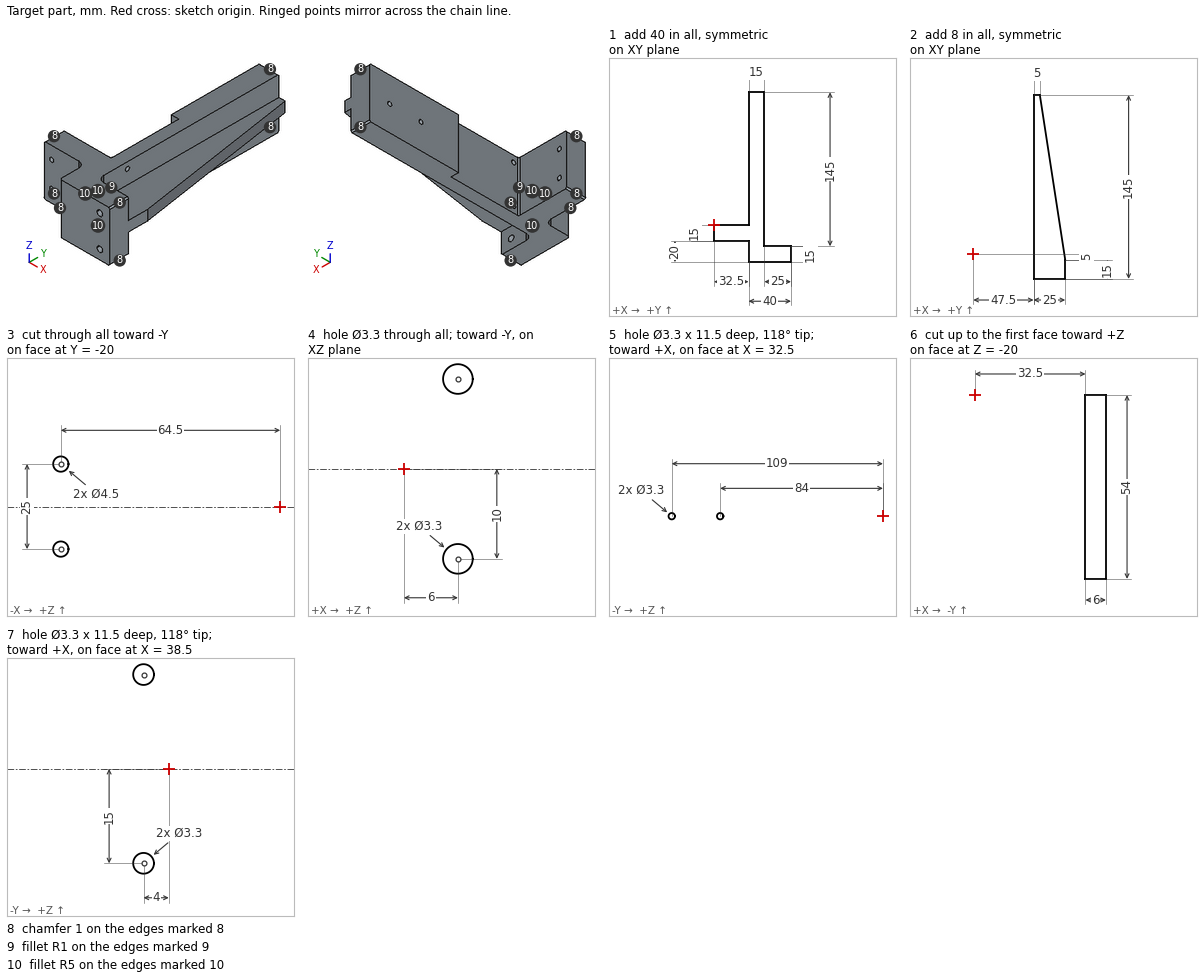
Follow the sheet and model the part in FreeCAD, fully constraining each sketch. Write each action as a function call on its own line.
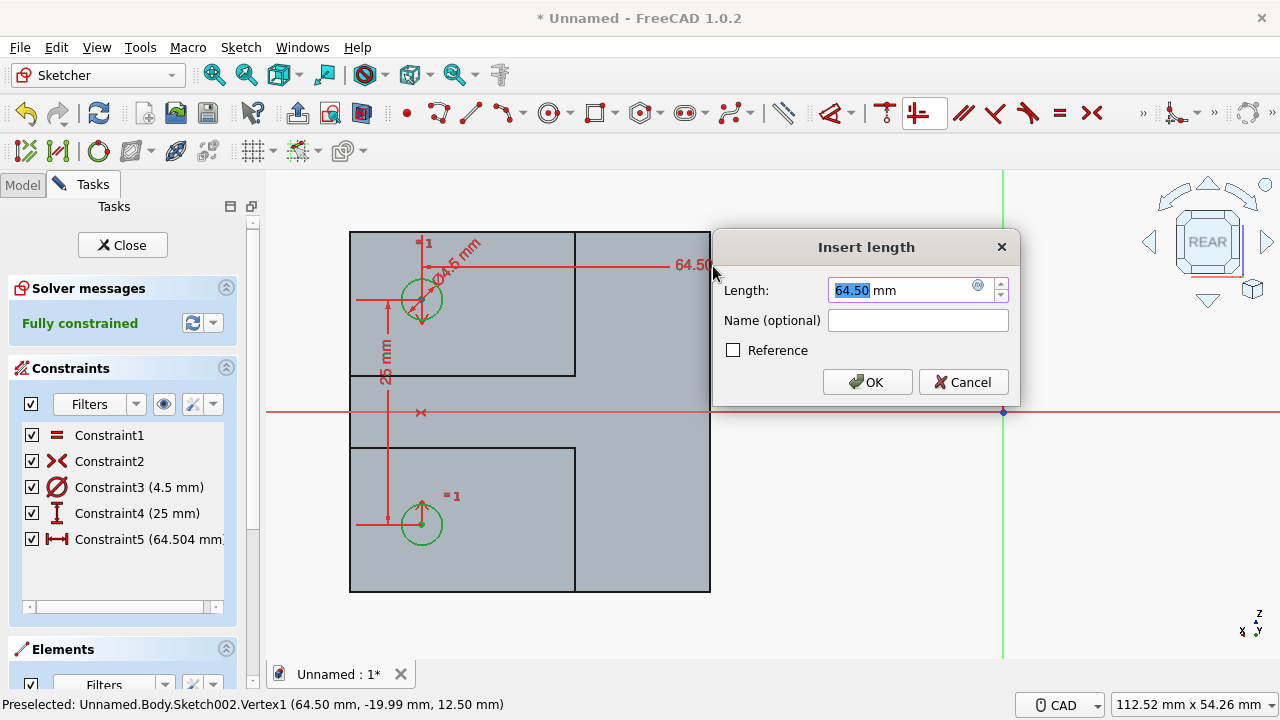
text(64.5)
key(Return)
key(Escape)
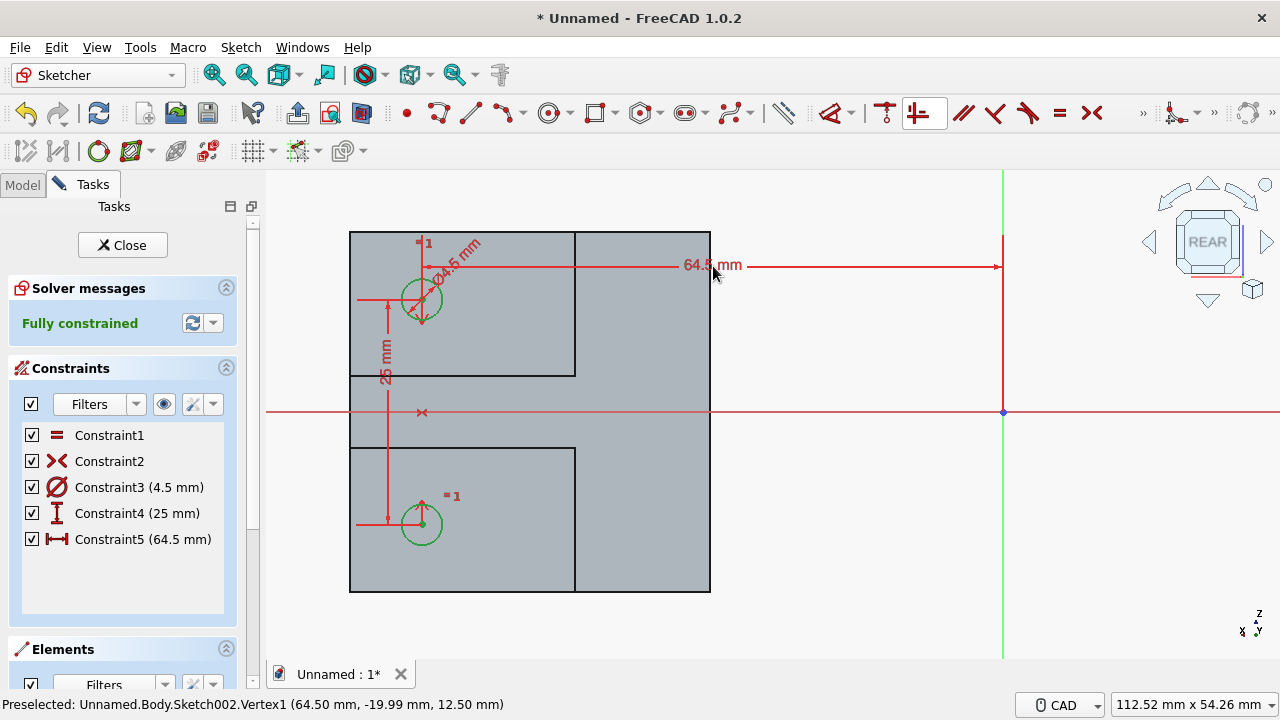
click(123, 245)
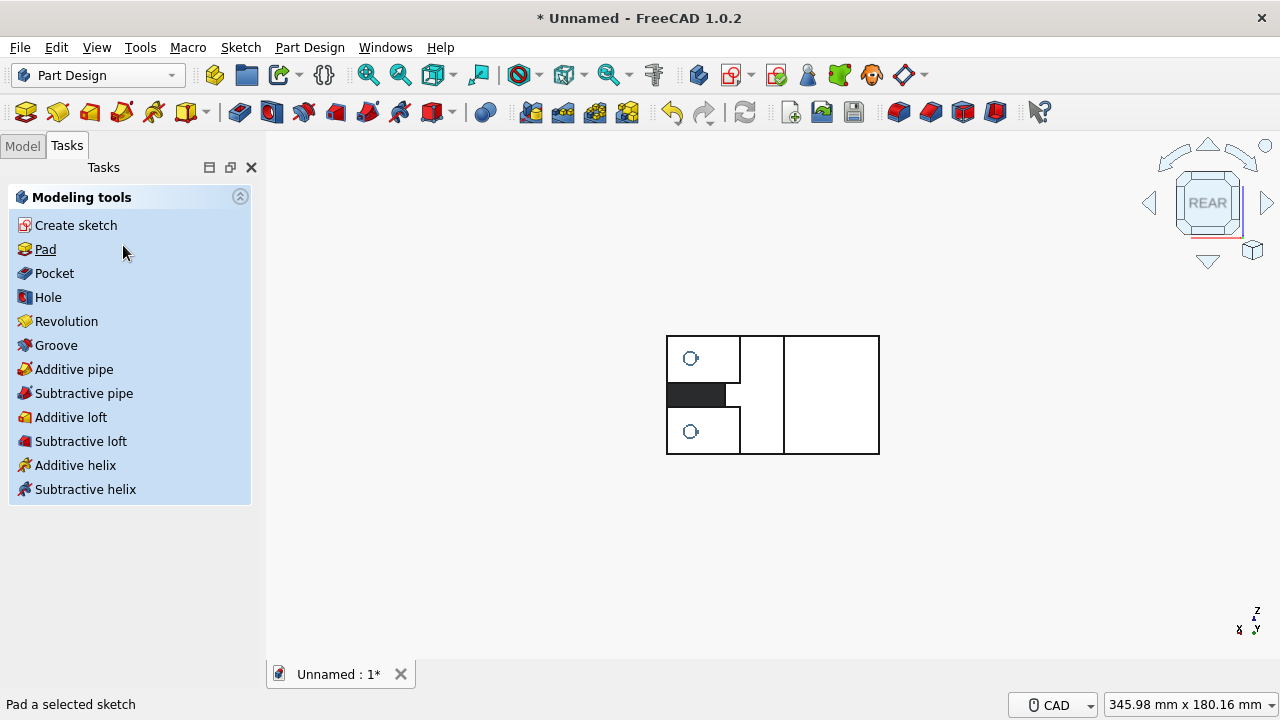
click(240, 112)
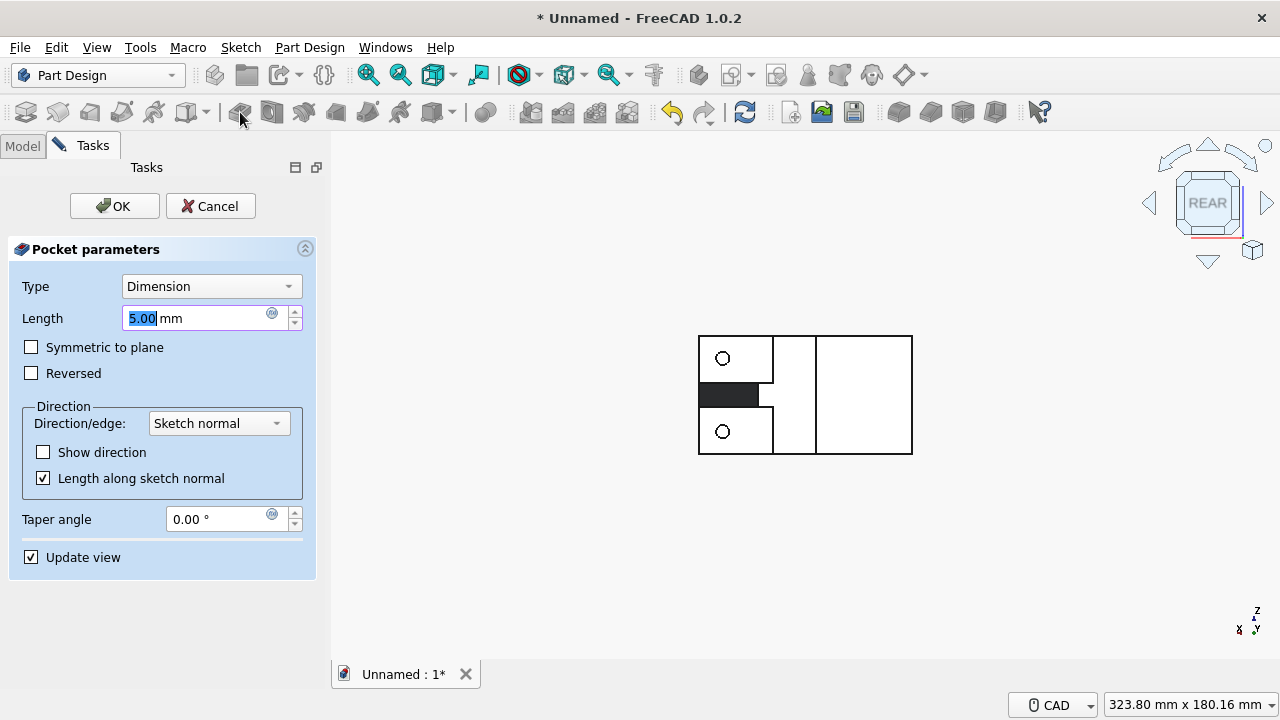
click(212, 286)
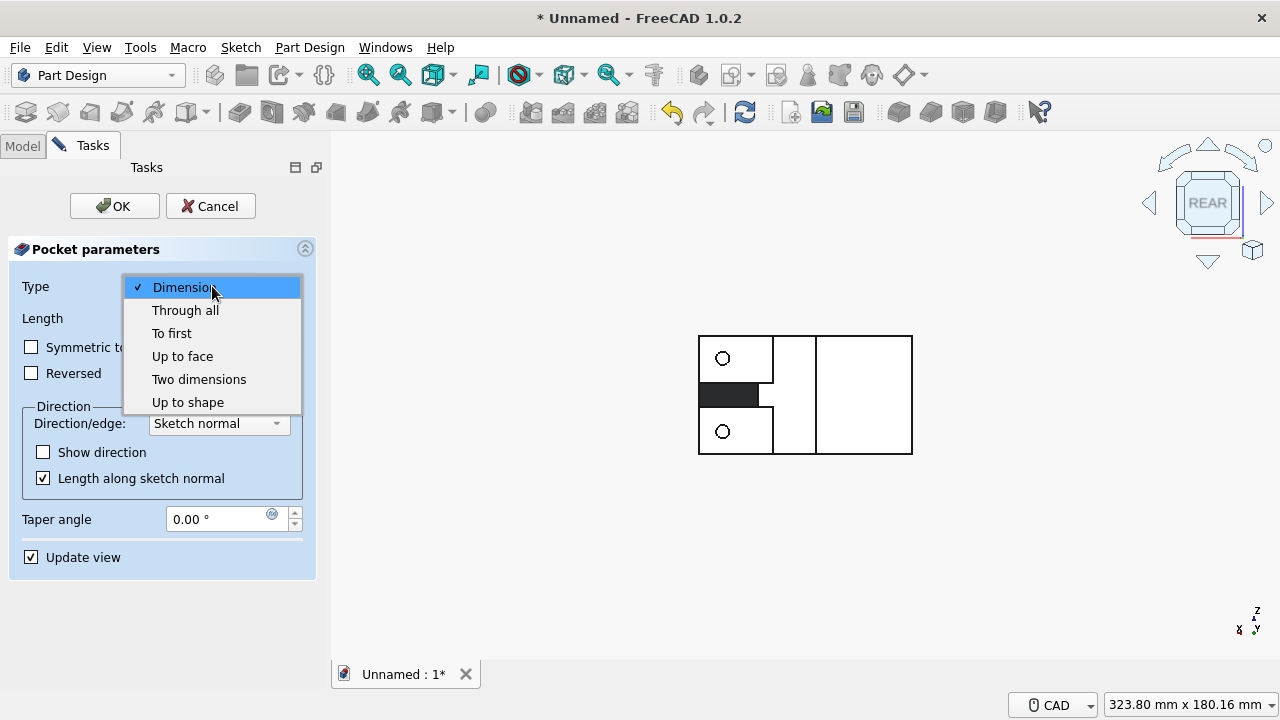
click(212, 310)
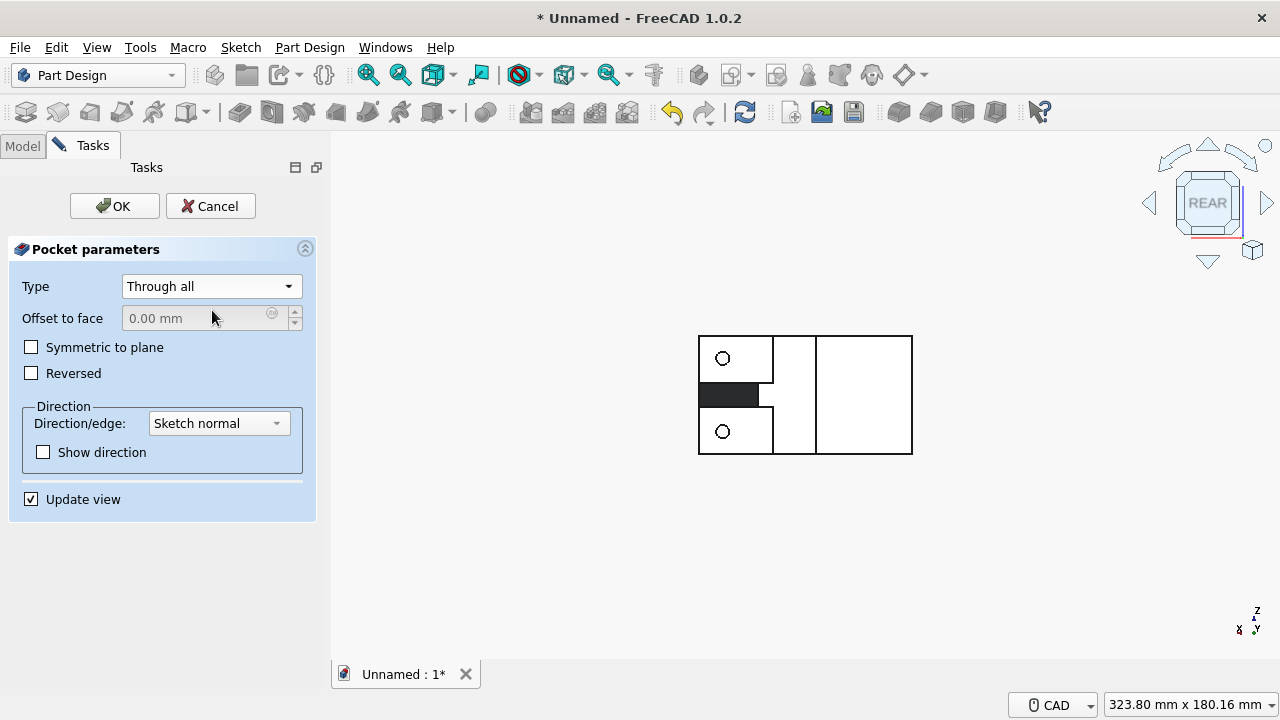
click(115, 206)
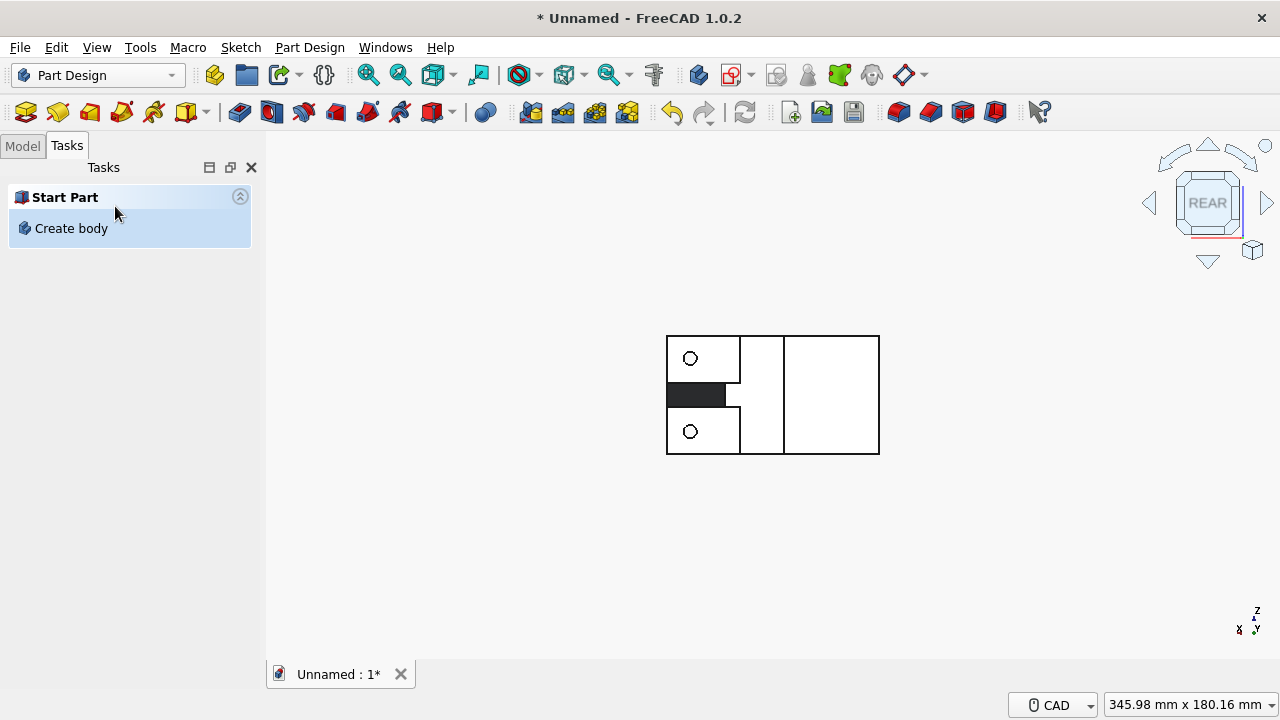
click(370, 76)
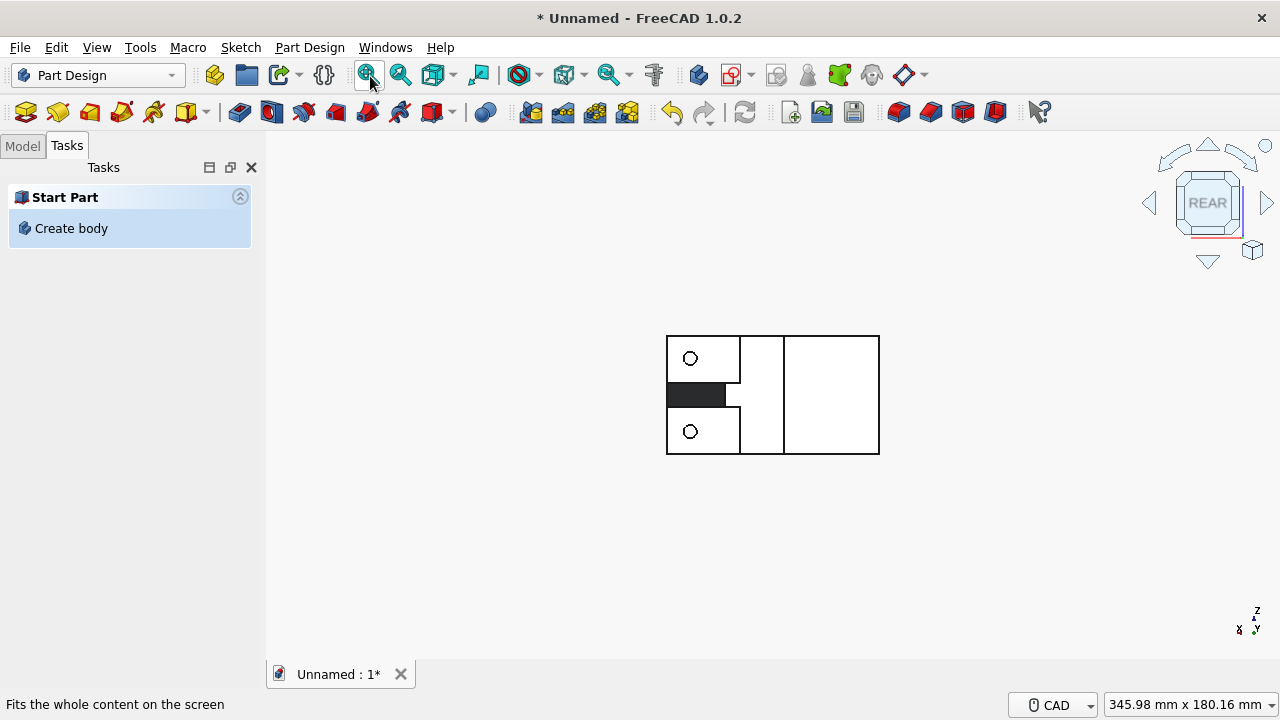
click(732, 76)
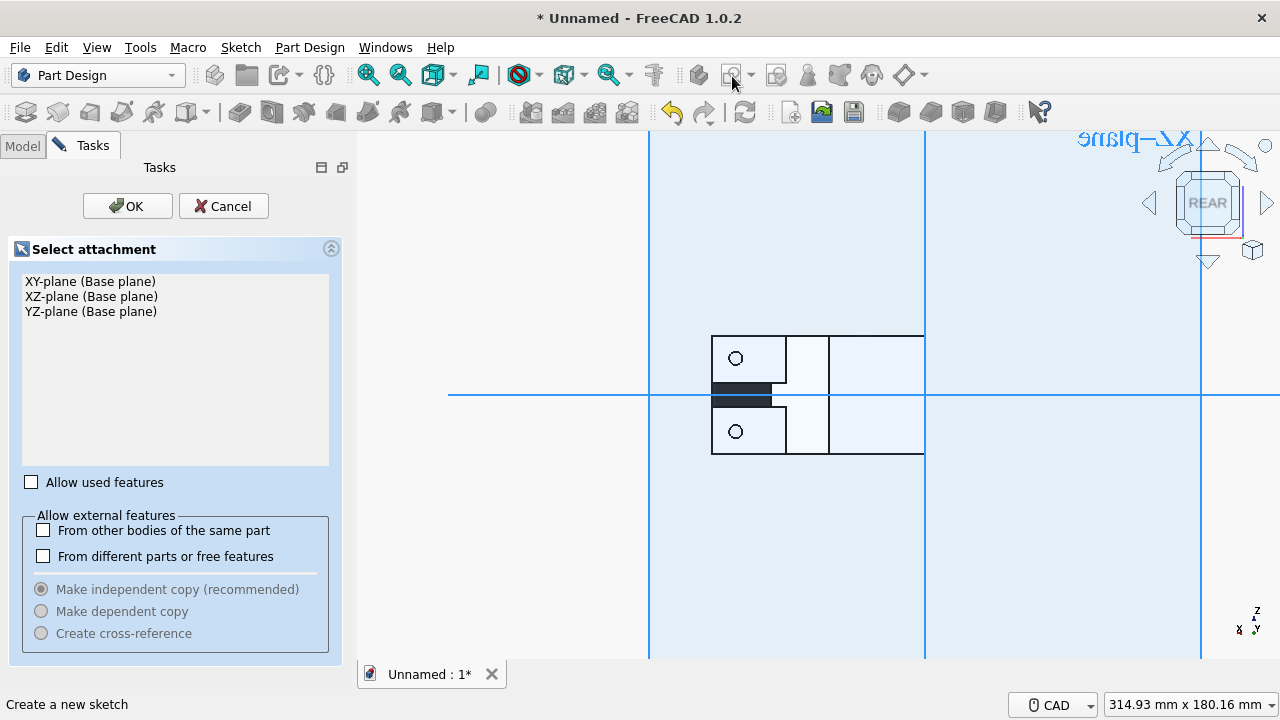
click(82, 296)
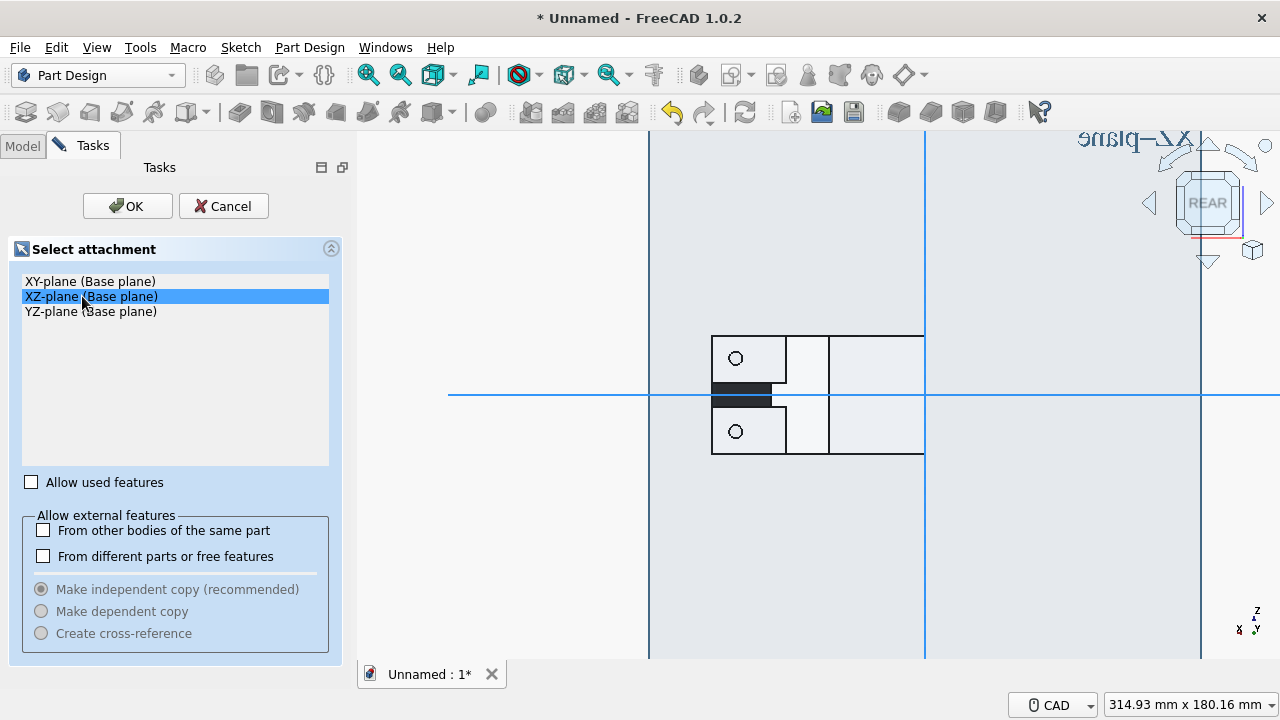
click(128, 206)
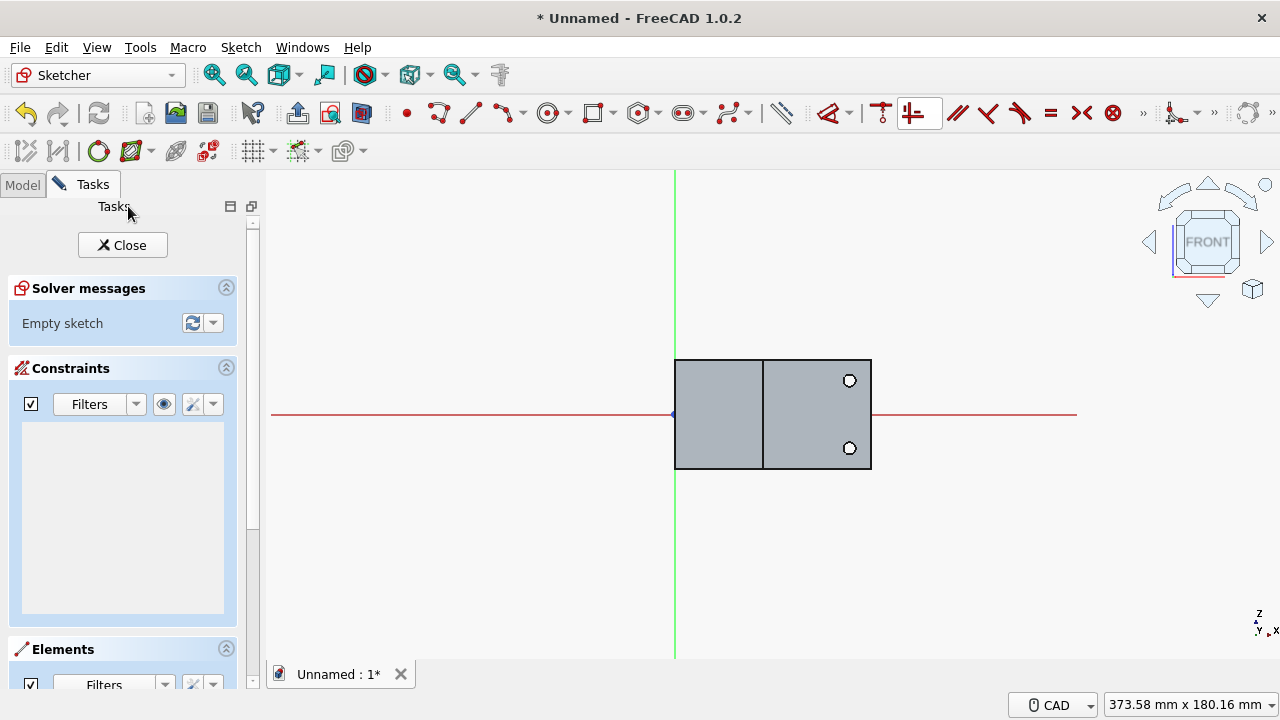
click(362, 114)